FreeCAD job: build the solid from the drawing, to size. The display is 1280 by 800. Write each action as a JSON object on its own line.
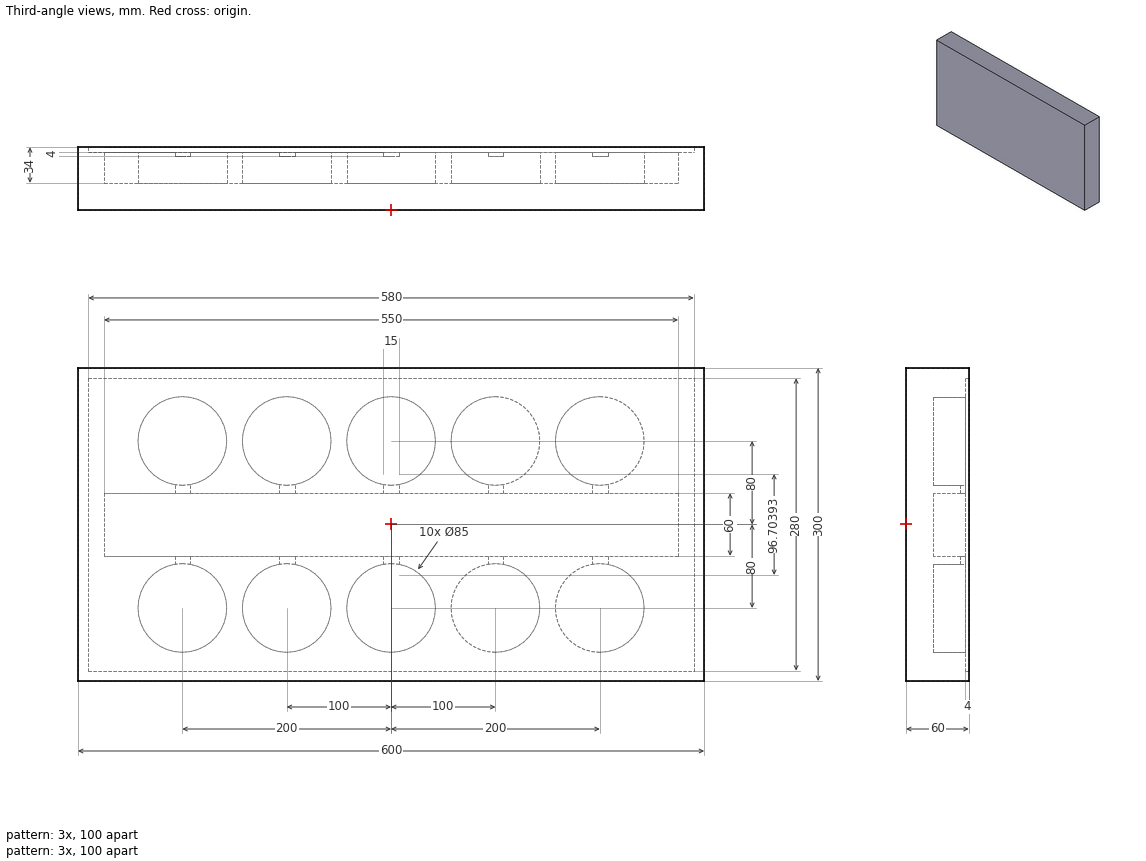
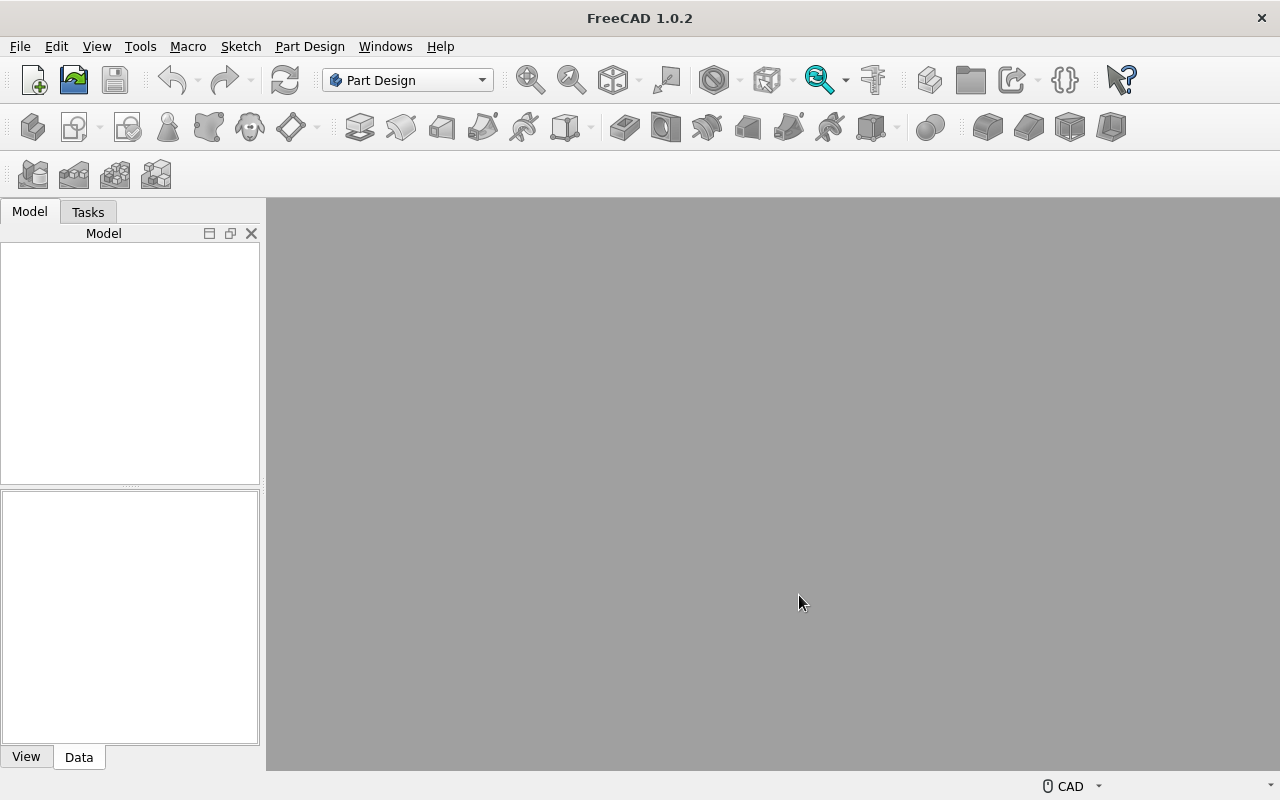
{"action": "left_click", "coordinate": [33, 80]}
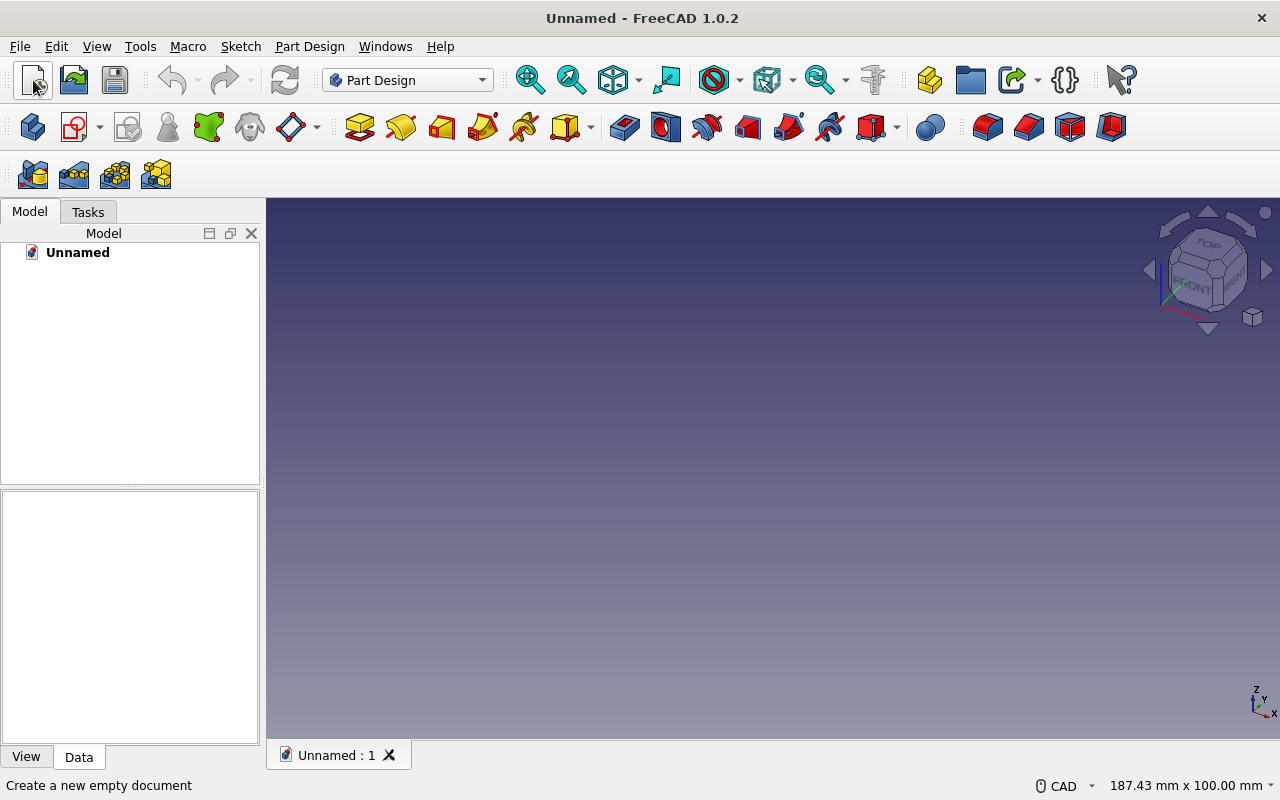
{"action": "left_click", "coordinate": [74, 128]}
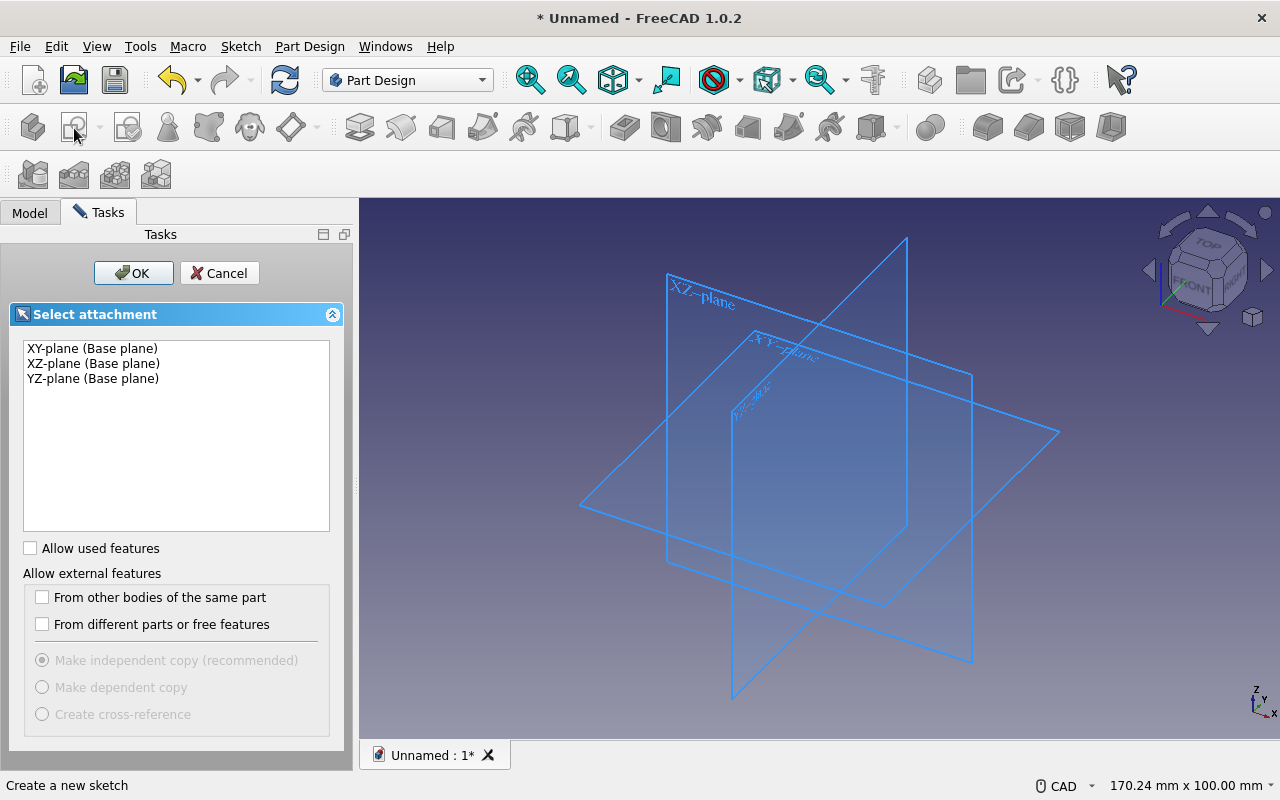
{"action": "left_click", "coordinate": [84, 364]}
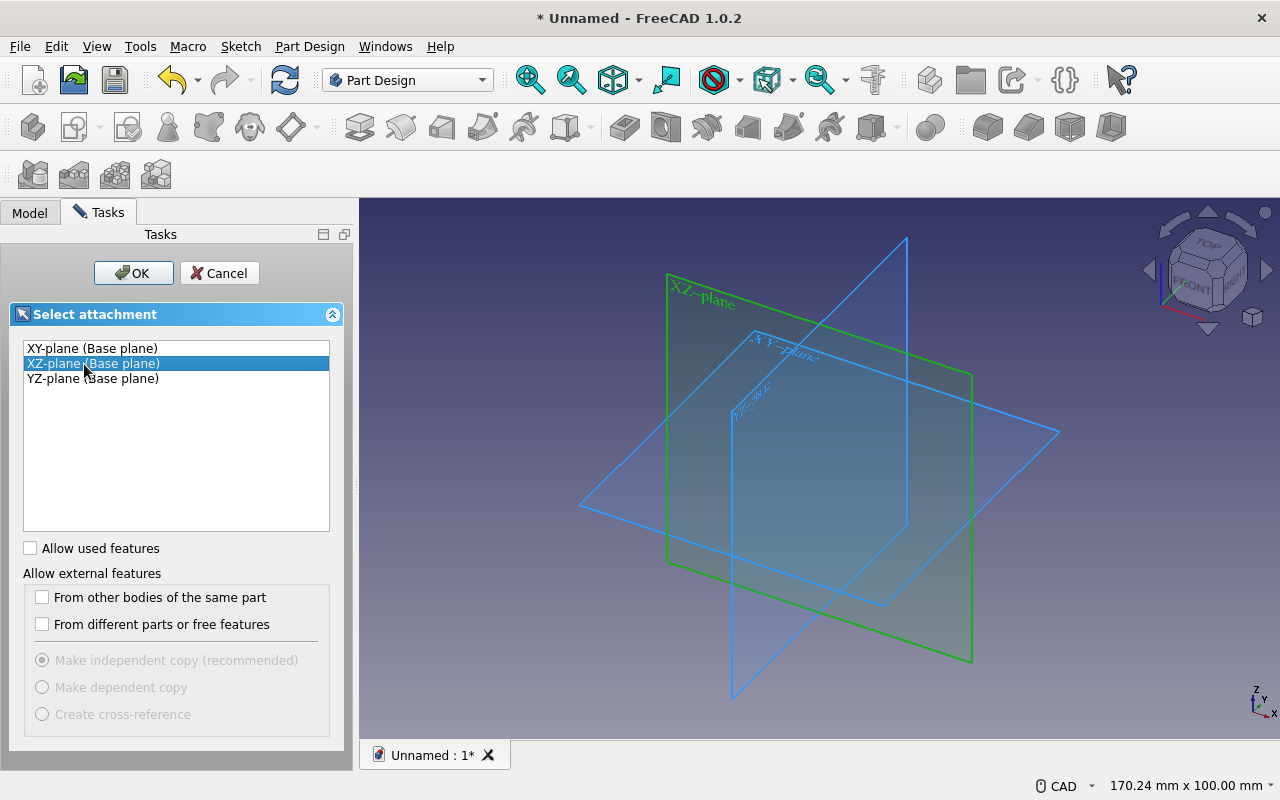
{"action": "left_click", "coordinate": [134, 273]}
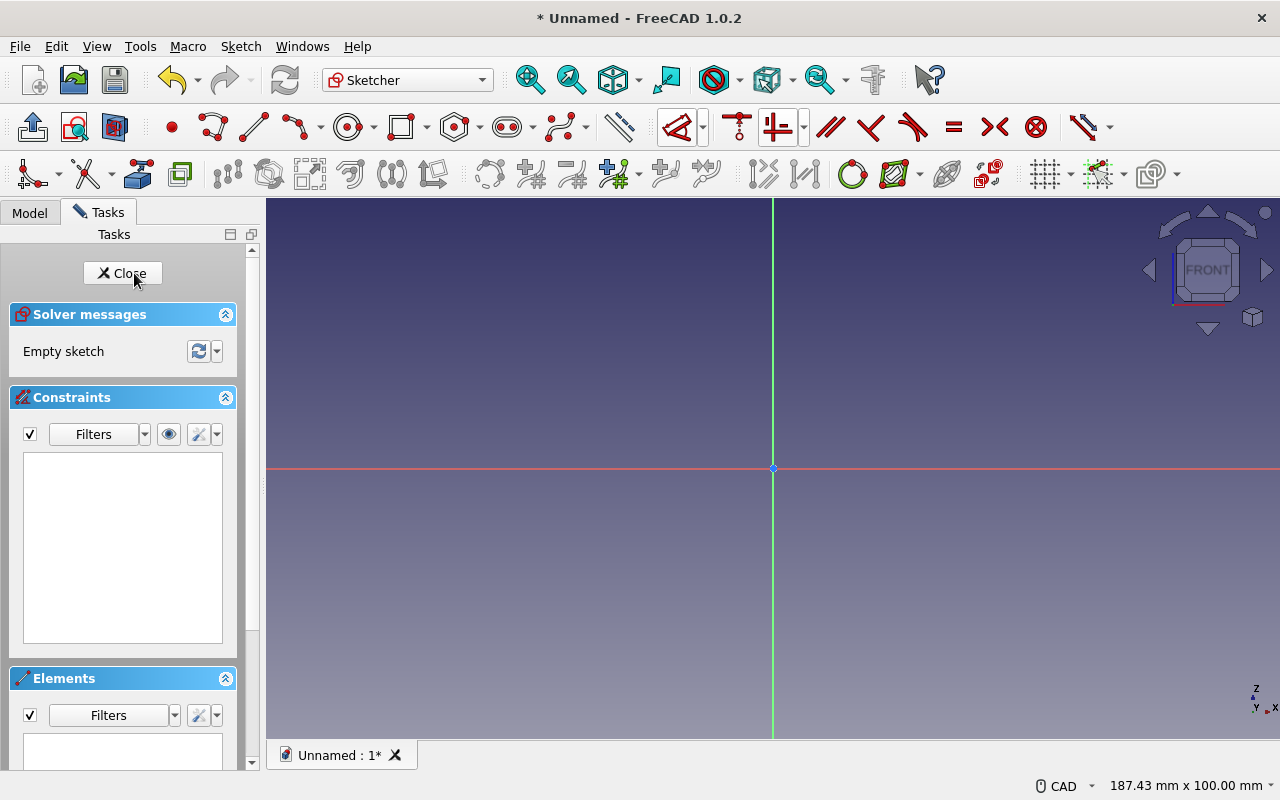
{"action": "scroll", "coordinate": [691, 468], "scroll_direction": "down", "scroll_amount": 9}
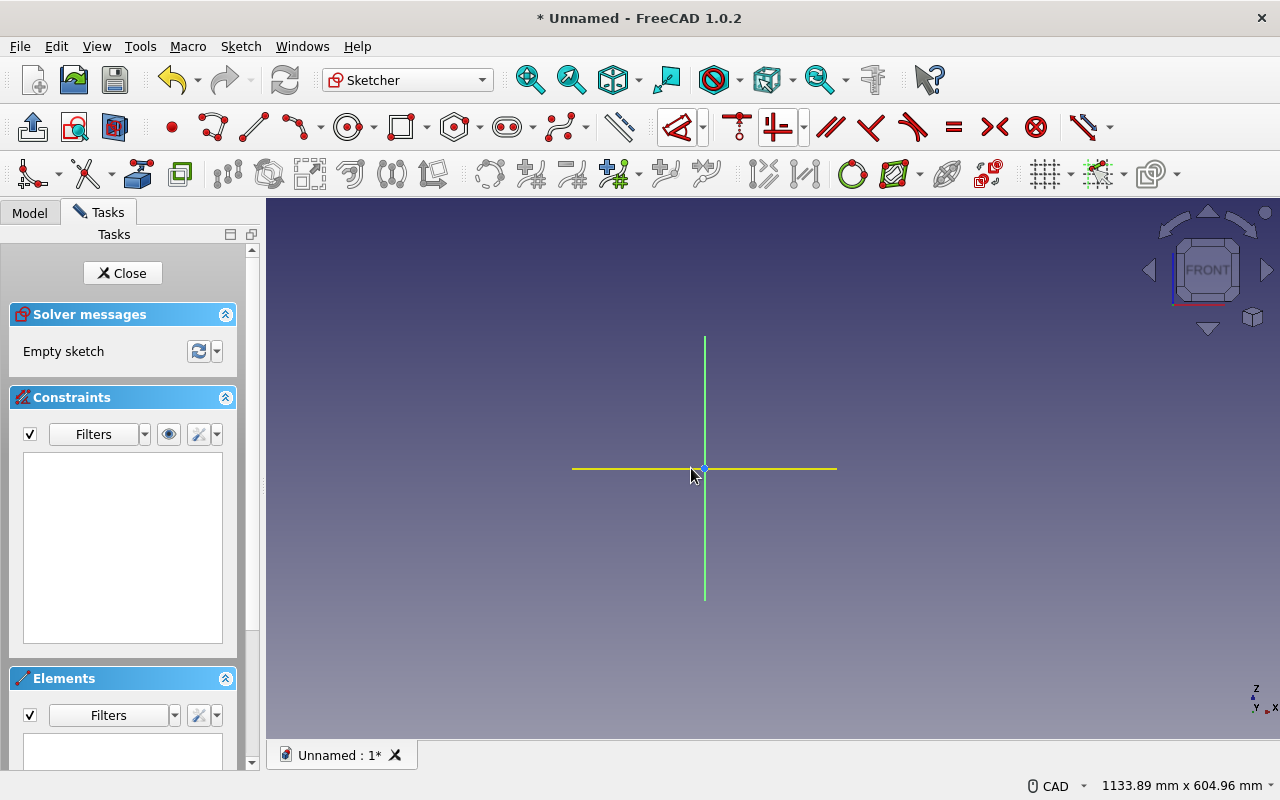
{"action": "left_click", "coordinate": [426, 128]}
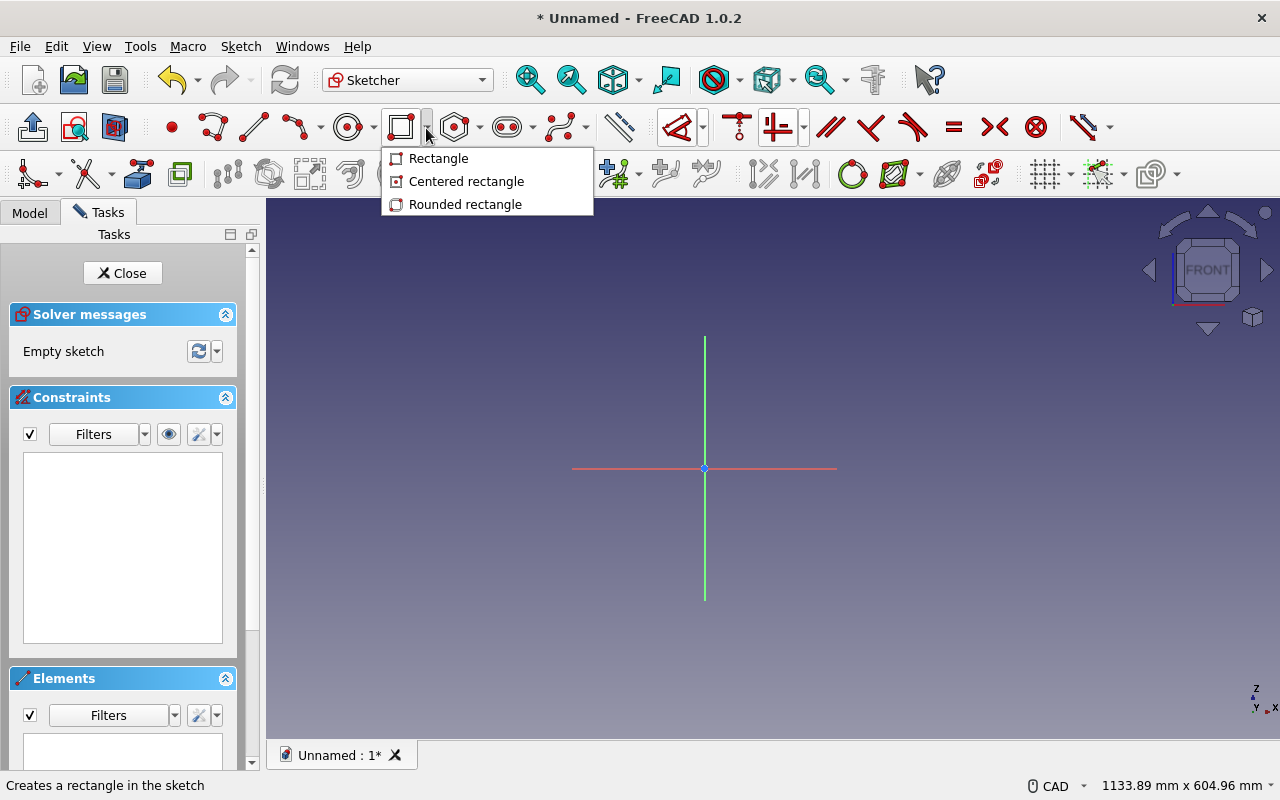
{"action": "left_click", "coordinate": [488, 182]}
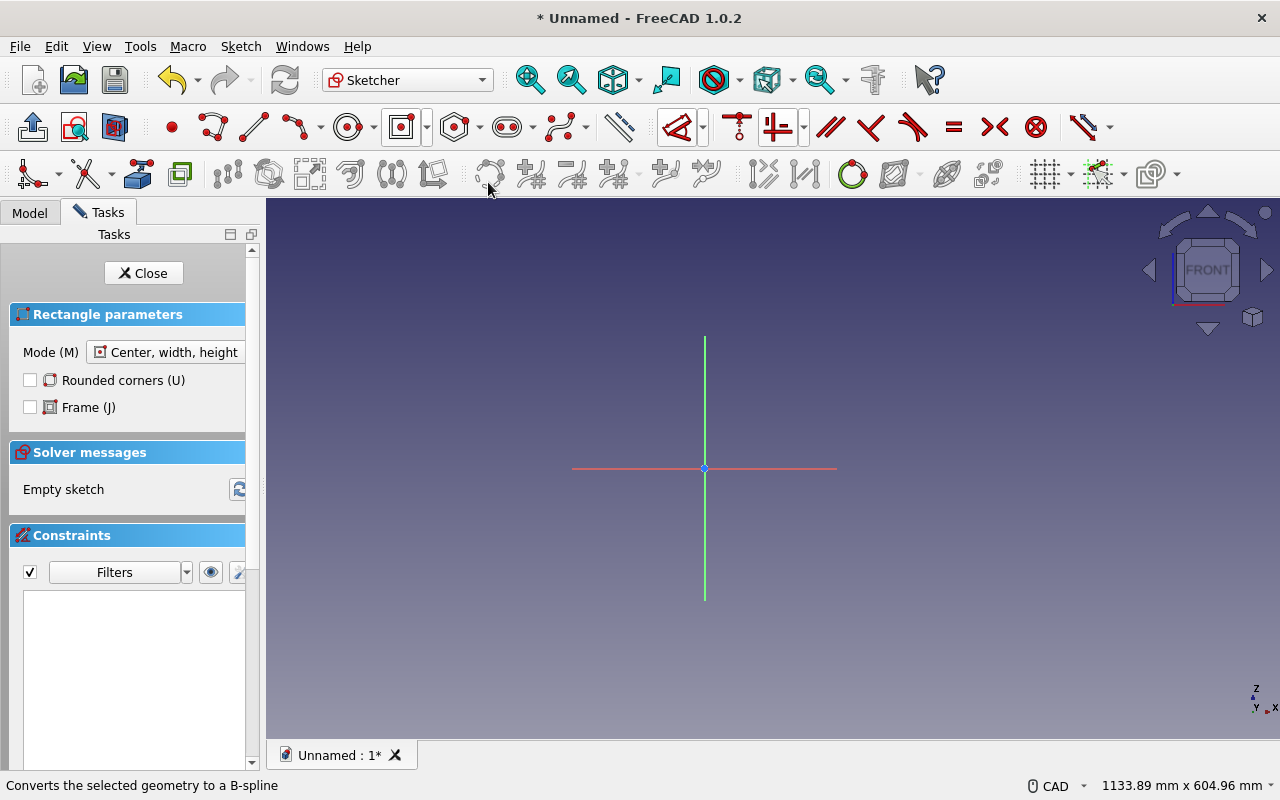
{"action": "left_click", "coordinate": [705, 468]}
{"action": "mouse_move", "coordinate": [973, 334]}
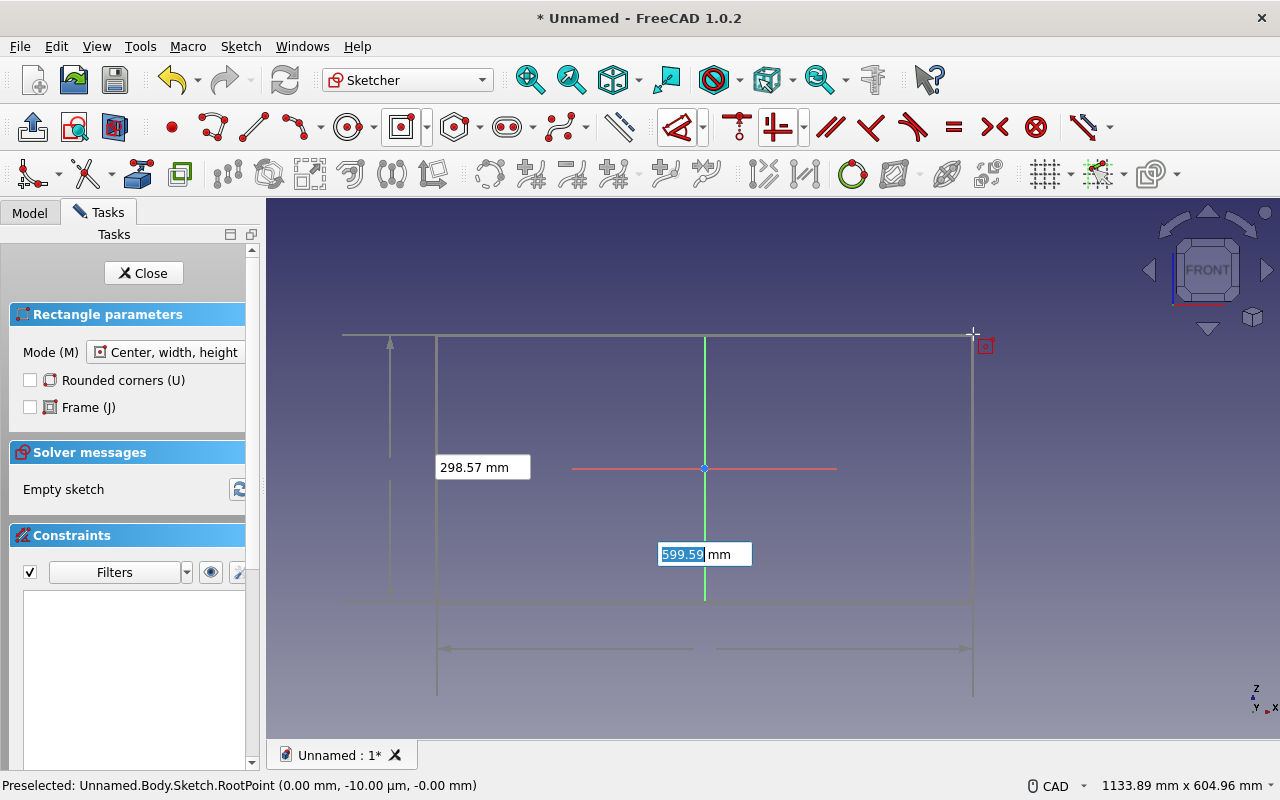
{"action": "type", "text": "600"}
{"action": "key", "text": "Tab"}
{"action": "type", "text": "300"}
{"action": "key", "text": "Return"}
{"action": "key", "text": "Escape"}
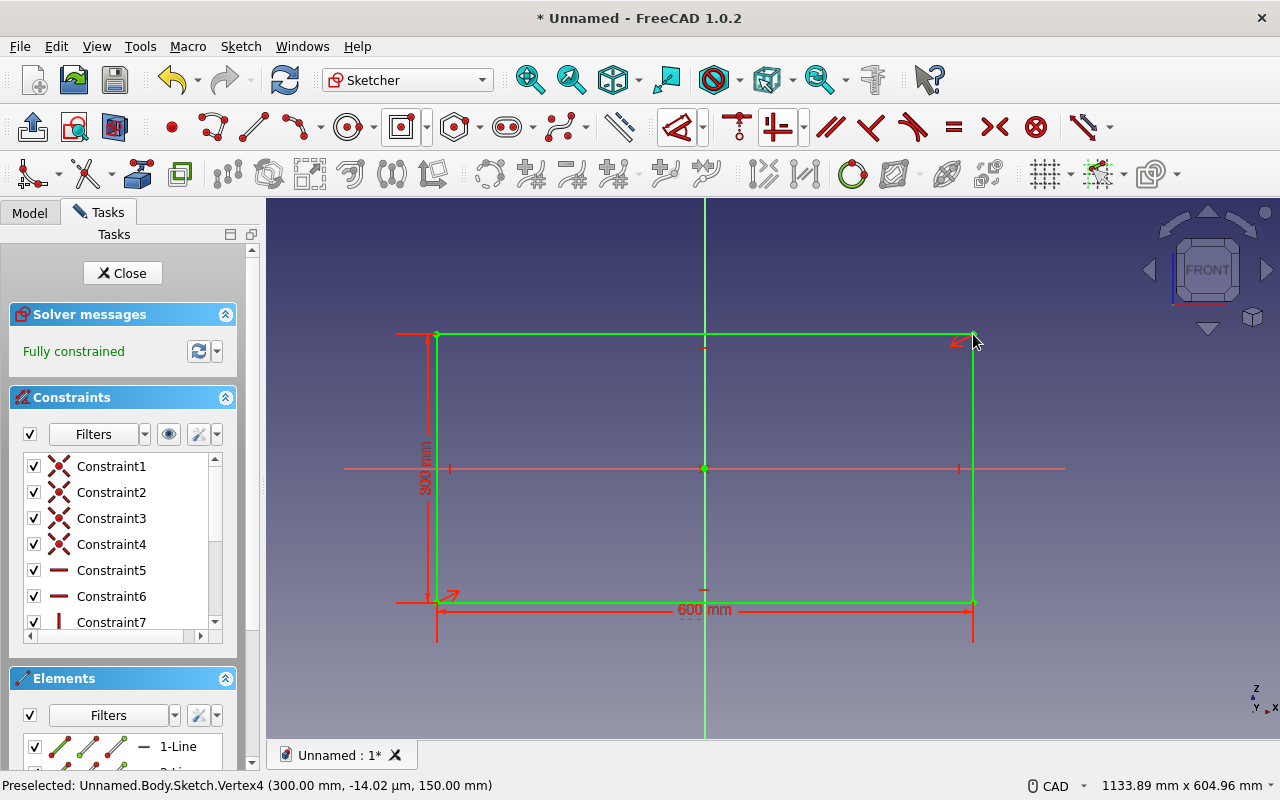
{"action": "left_click", "coordinate": [123, 273]}